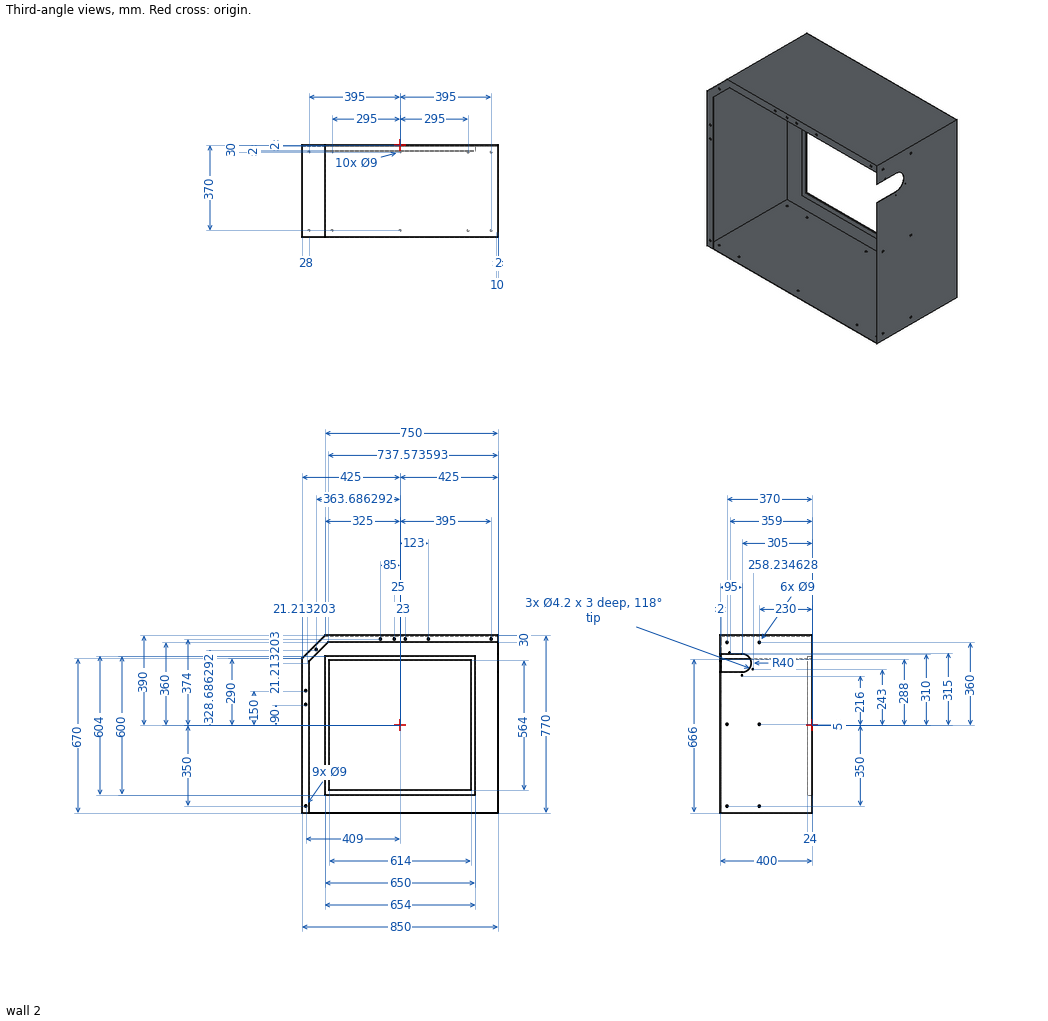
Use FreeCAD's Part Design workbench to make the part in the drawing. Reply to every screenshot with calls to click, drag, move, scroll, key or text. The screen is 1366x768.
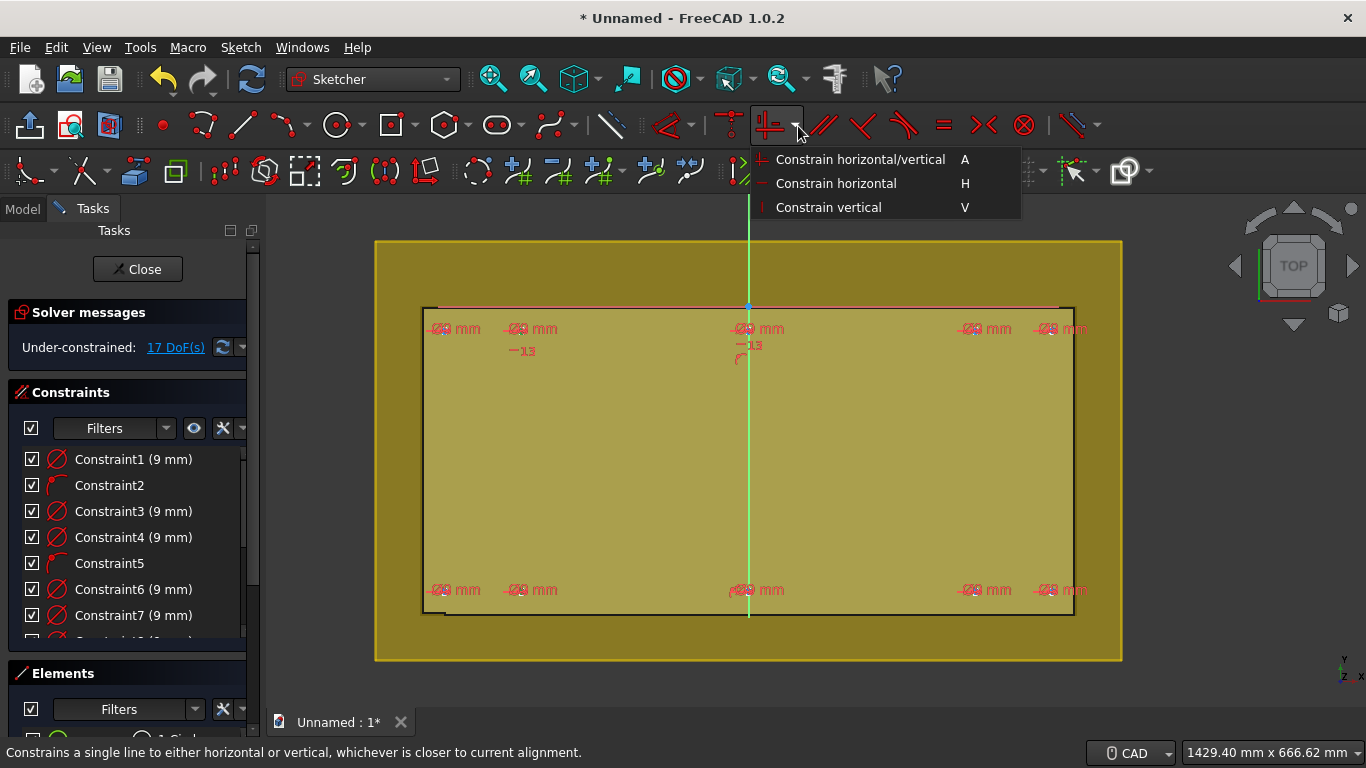
click(886, 207)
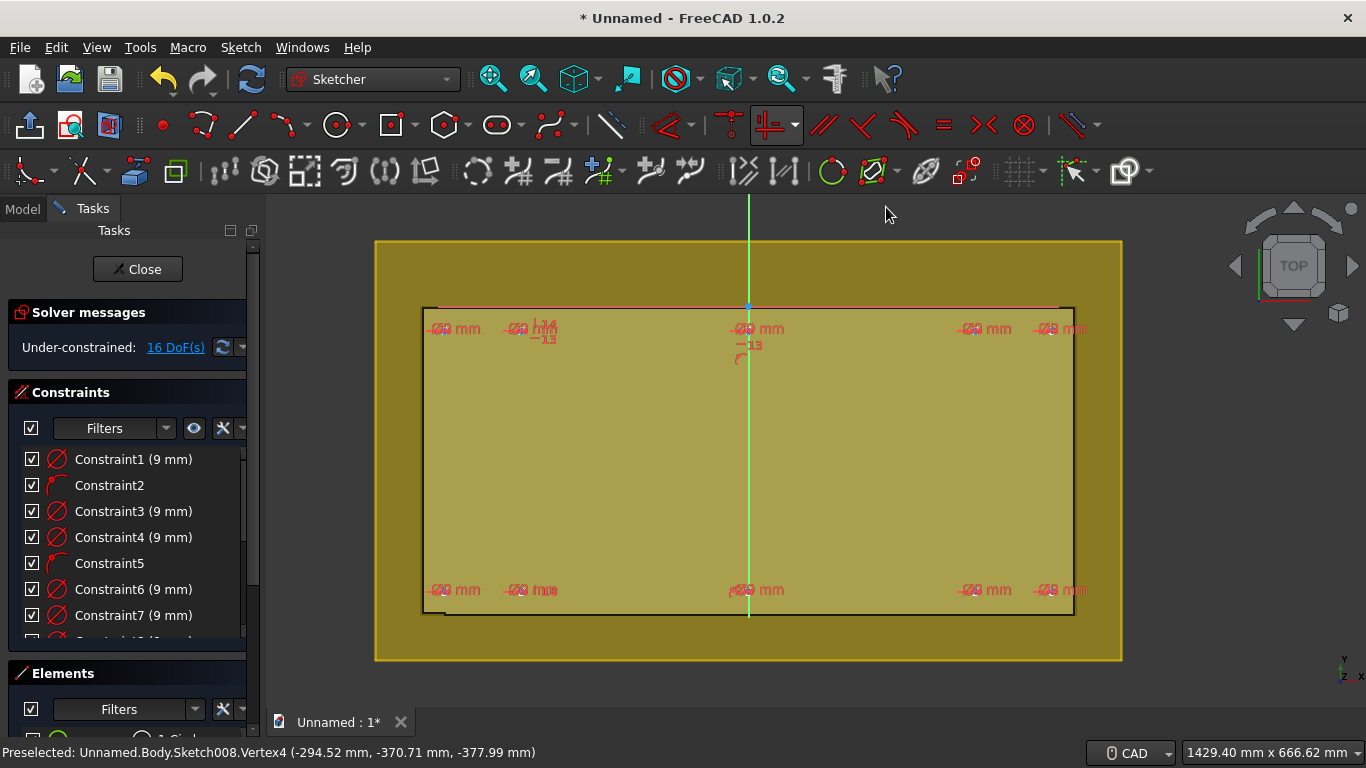
click(749, 592)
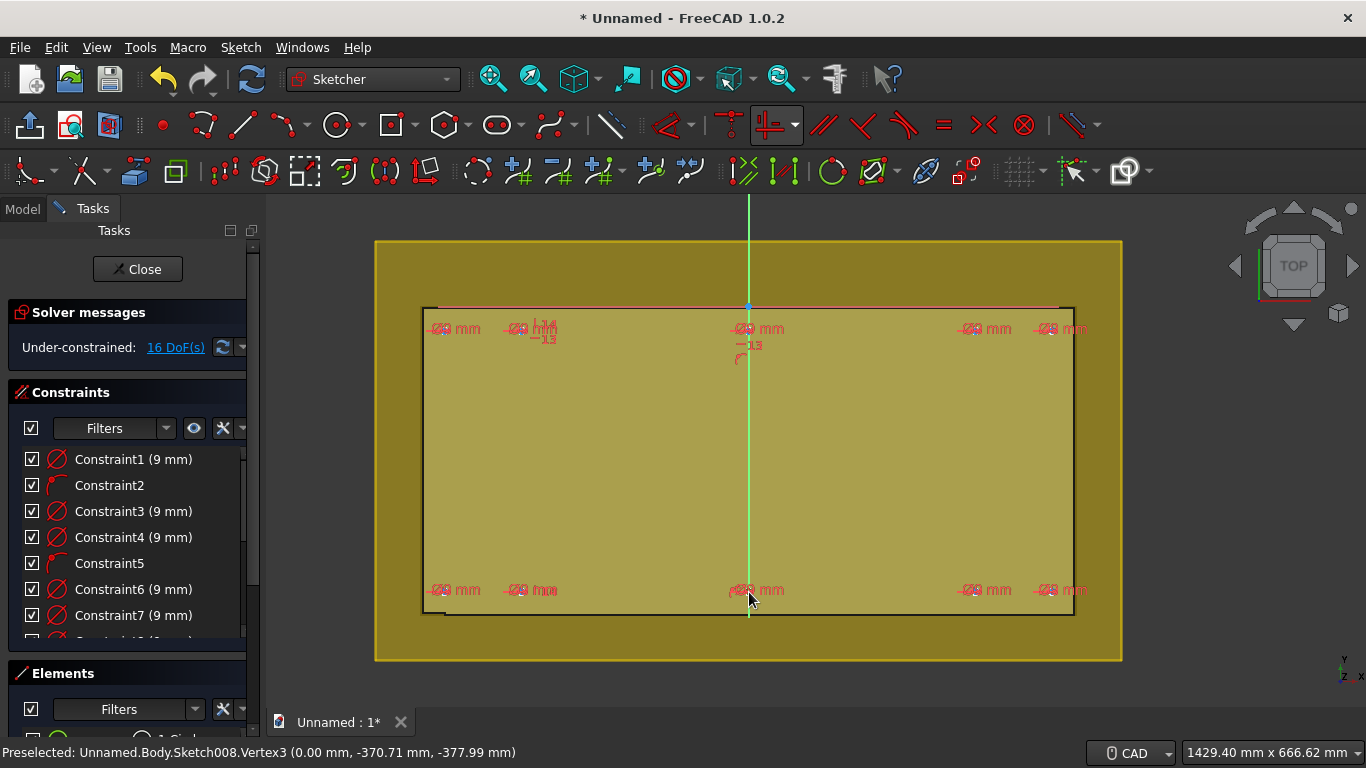
click(522, 592)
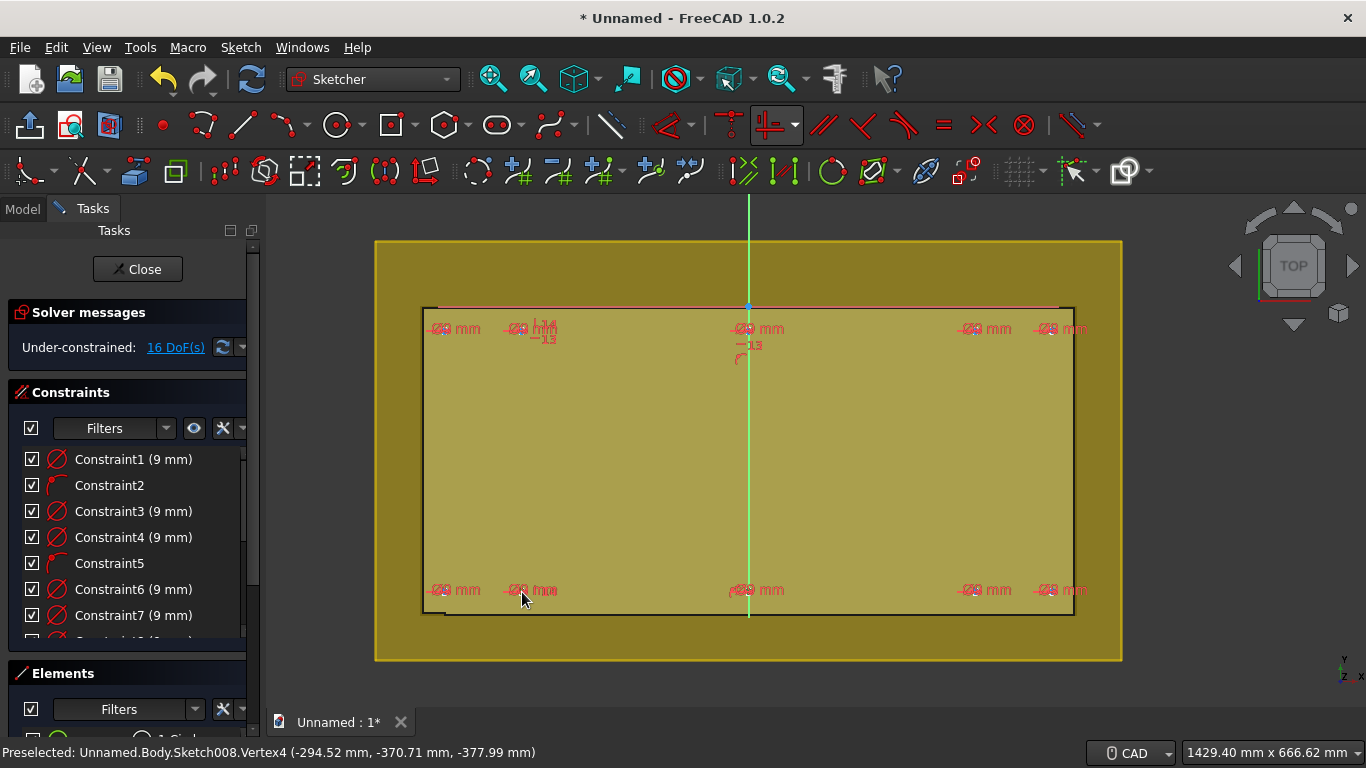
click(798, 126)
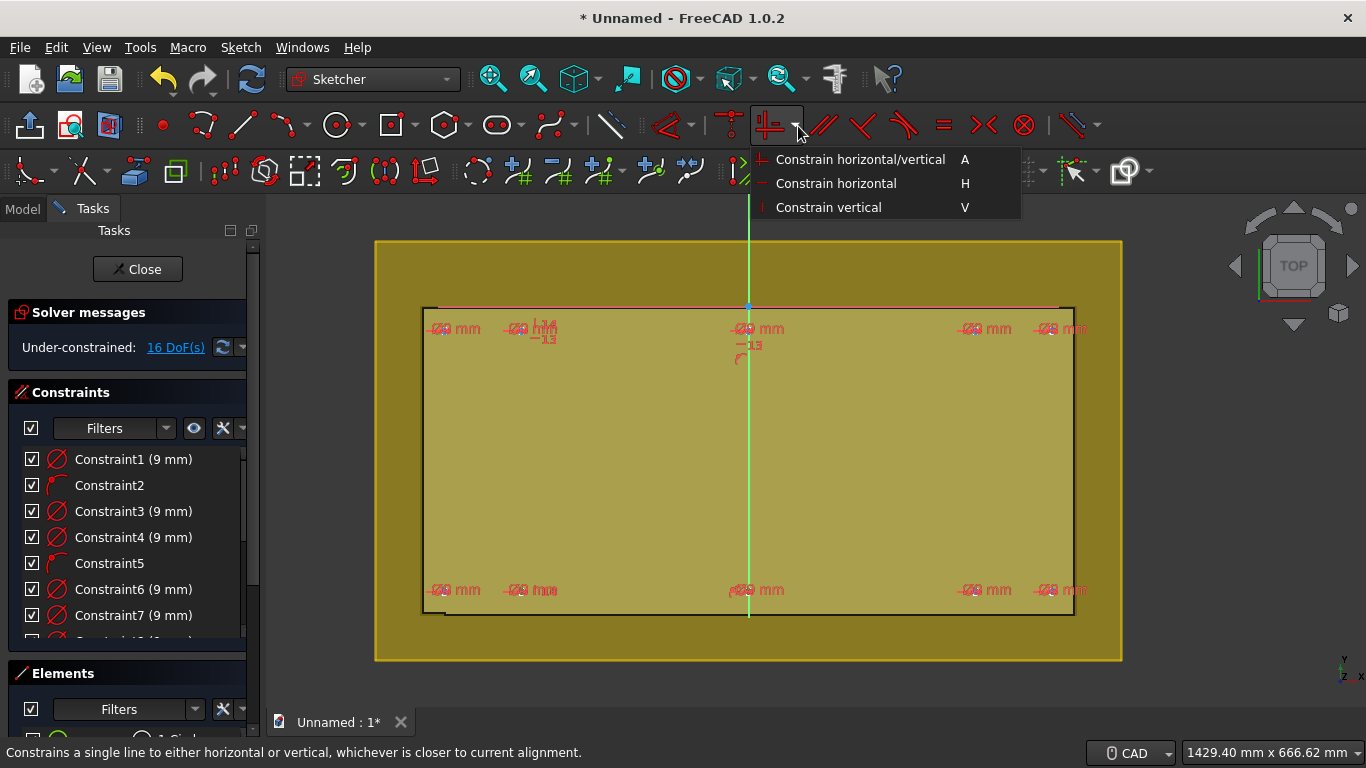
click(886, 183)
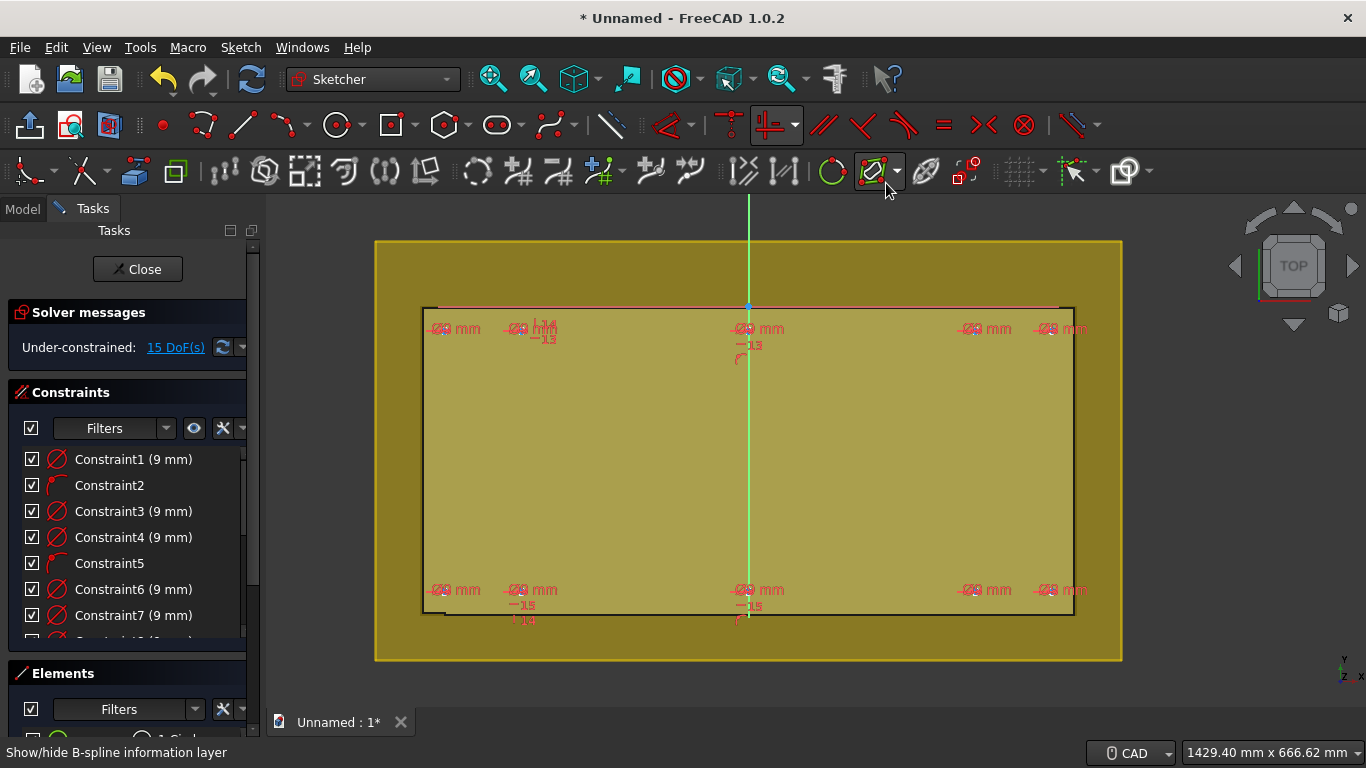
click(522, 331)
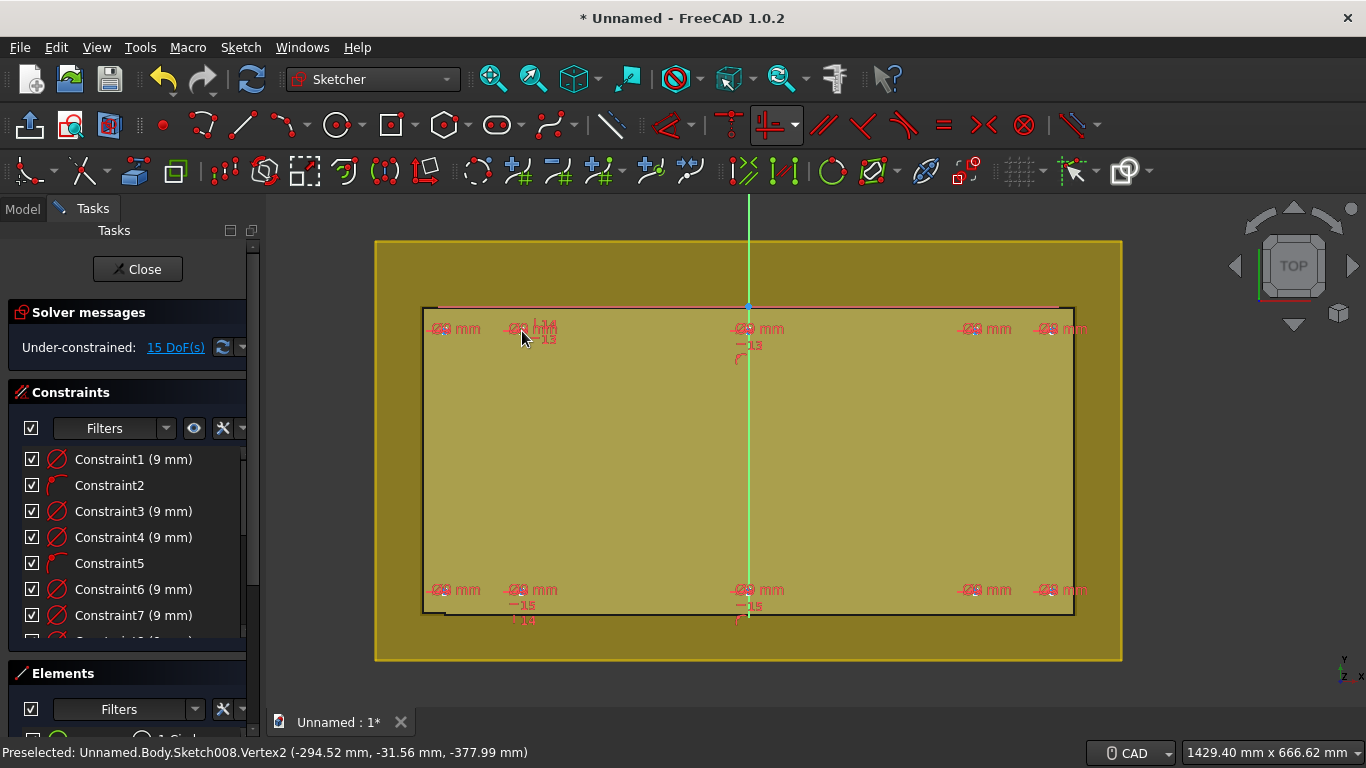
click(445, 331)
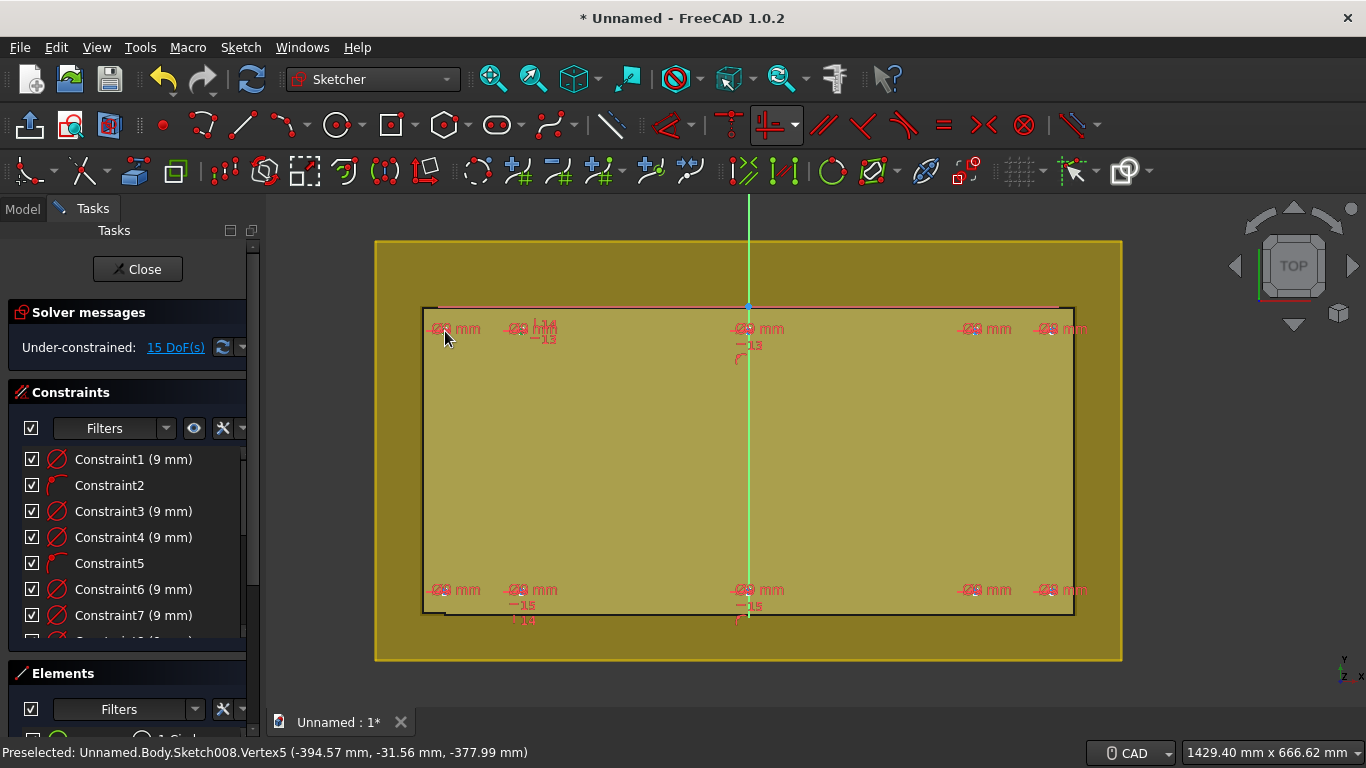
click(798, 126)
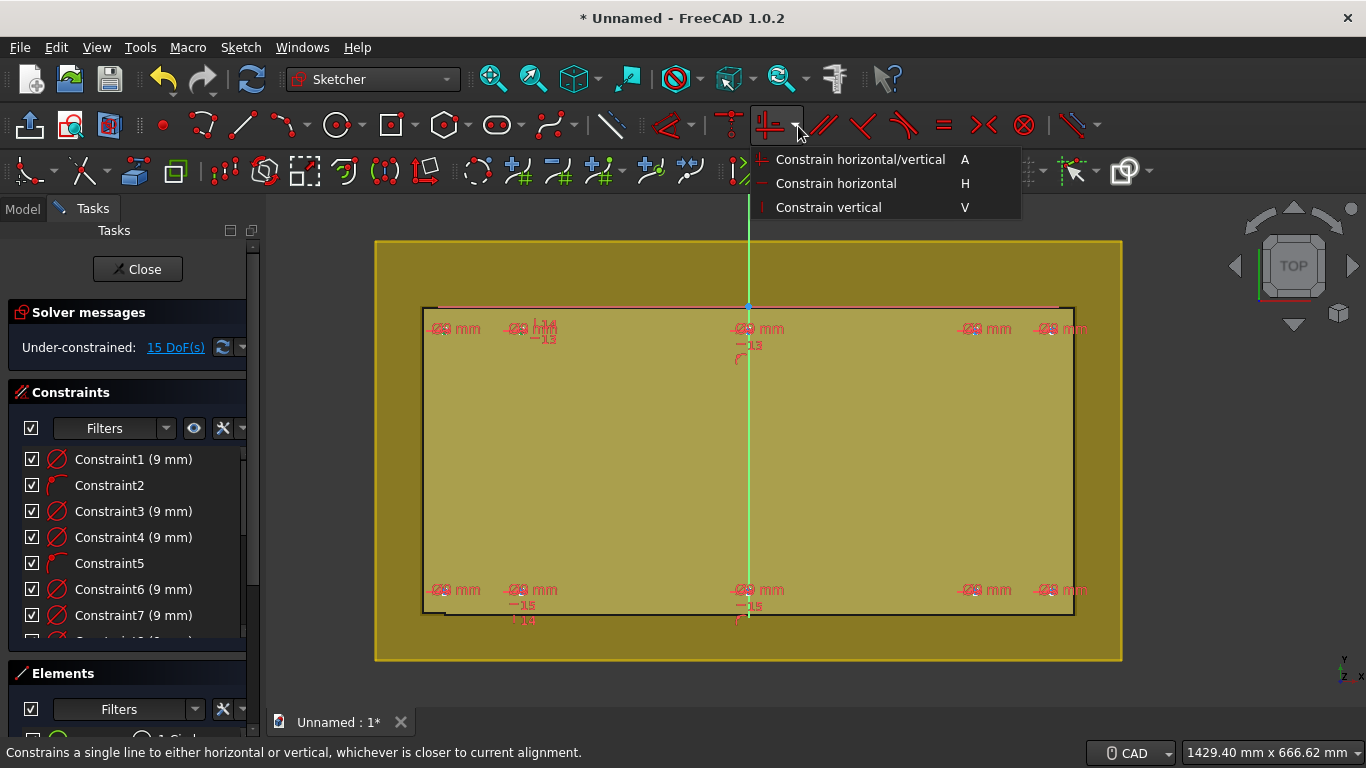
click(886, 183)